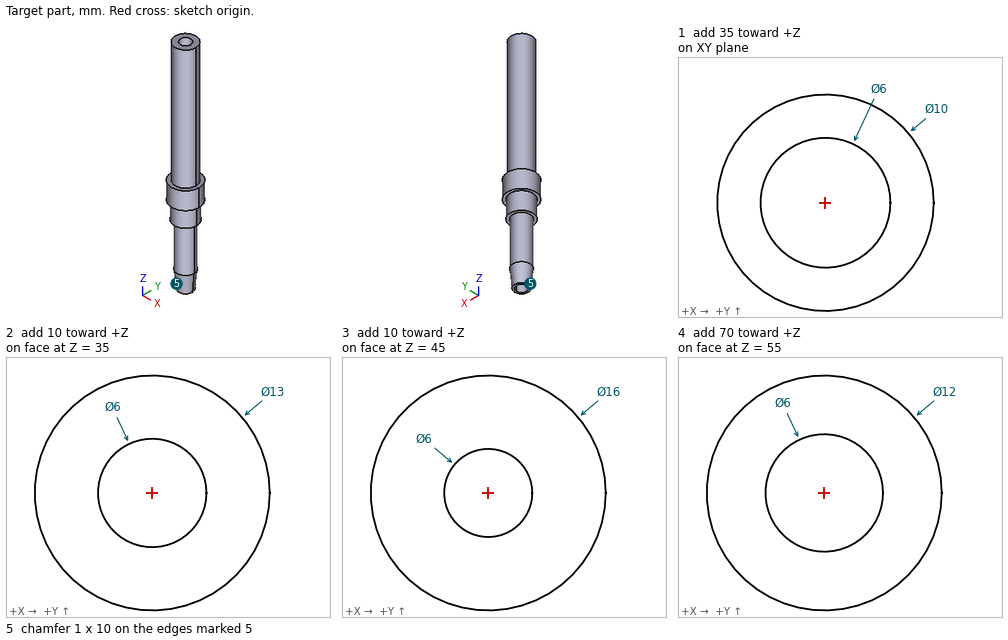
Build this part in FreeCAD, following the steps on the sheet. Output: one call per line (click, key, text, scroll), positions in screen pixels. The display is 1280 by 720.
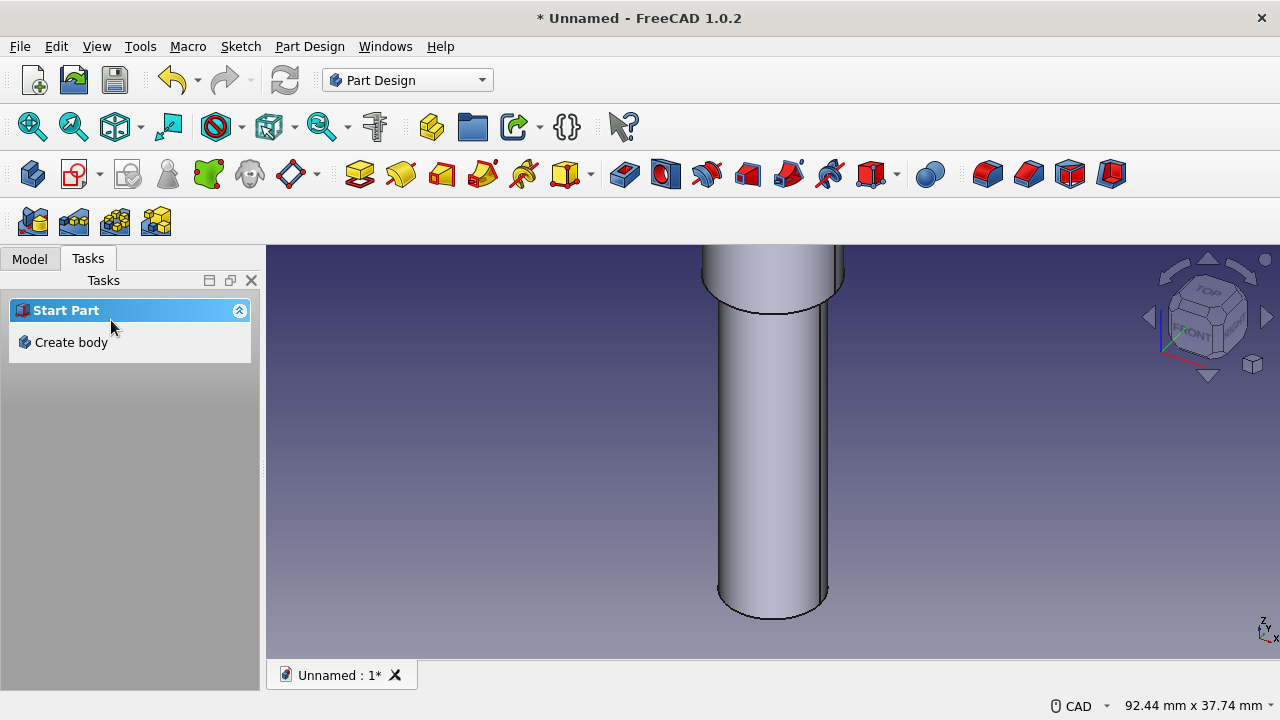
click(33, 128)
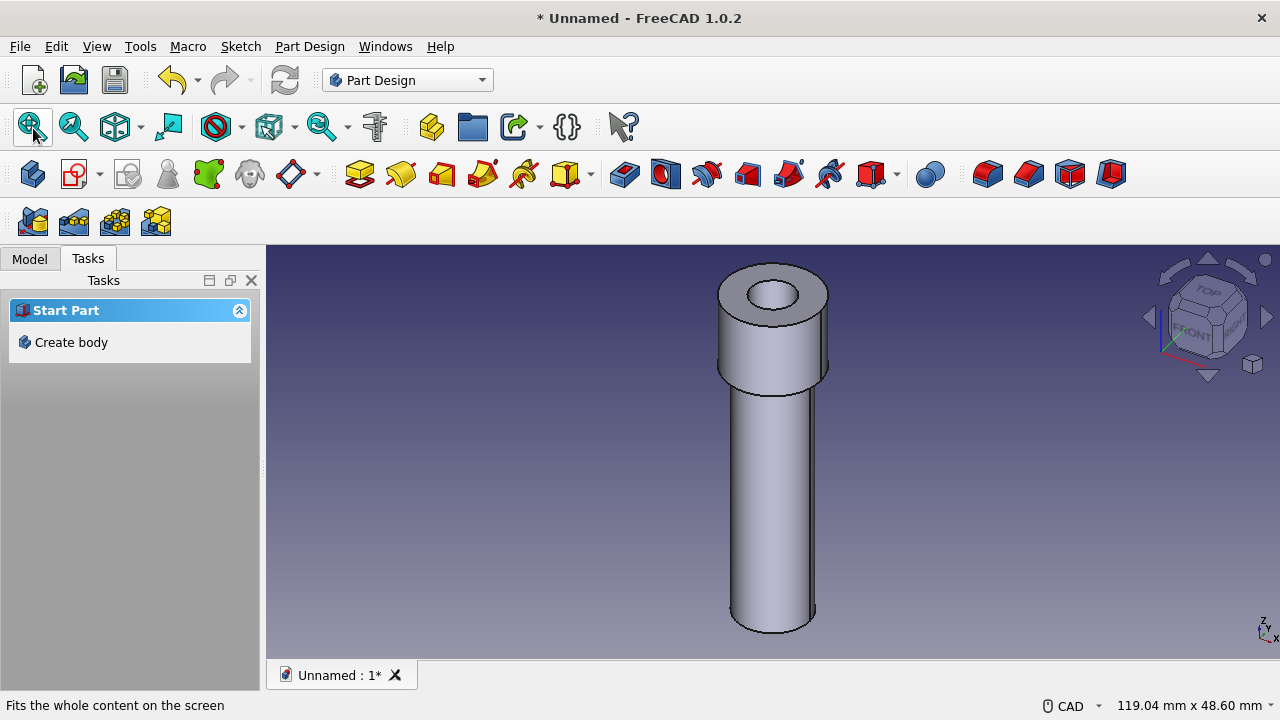
click(816, 287)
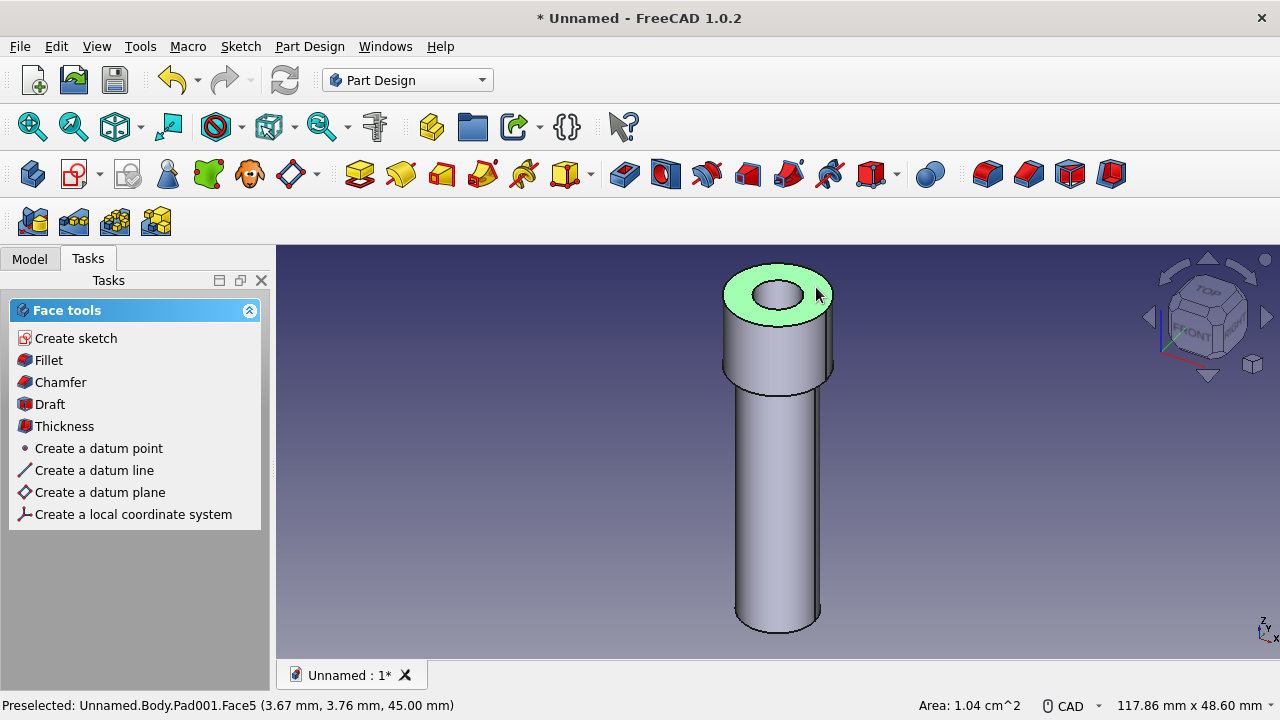
click(74, 174)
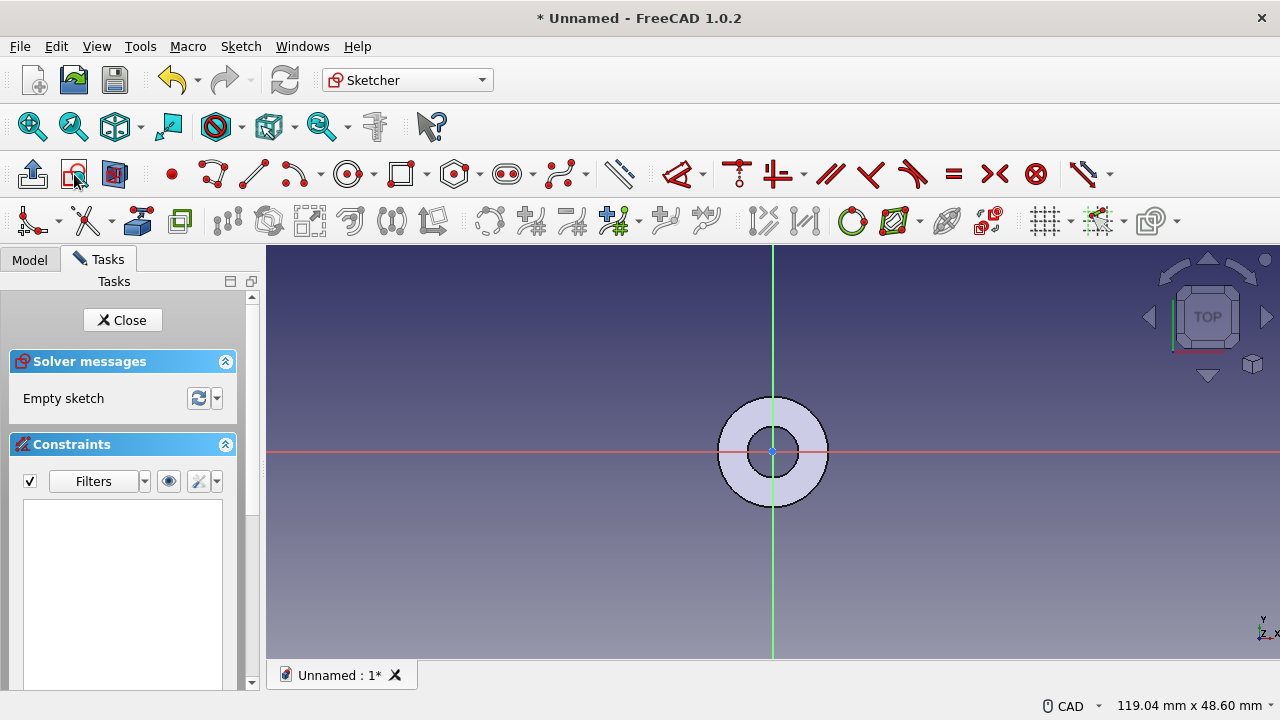
scroll(856, 452, up, 3)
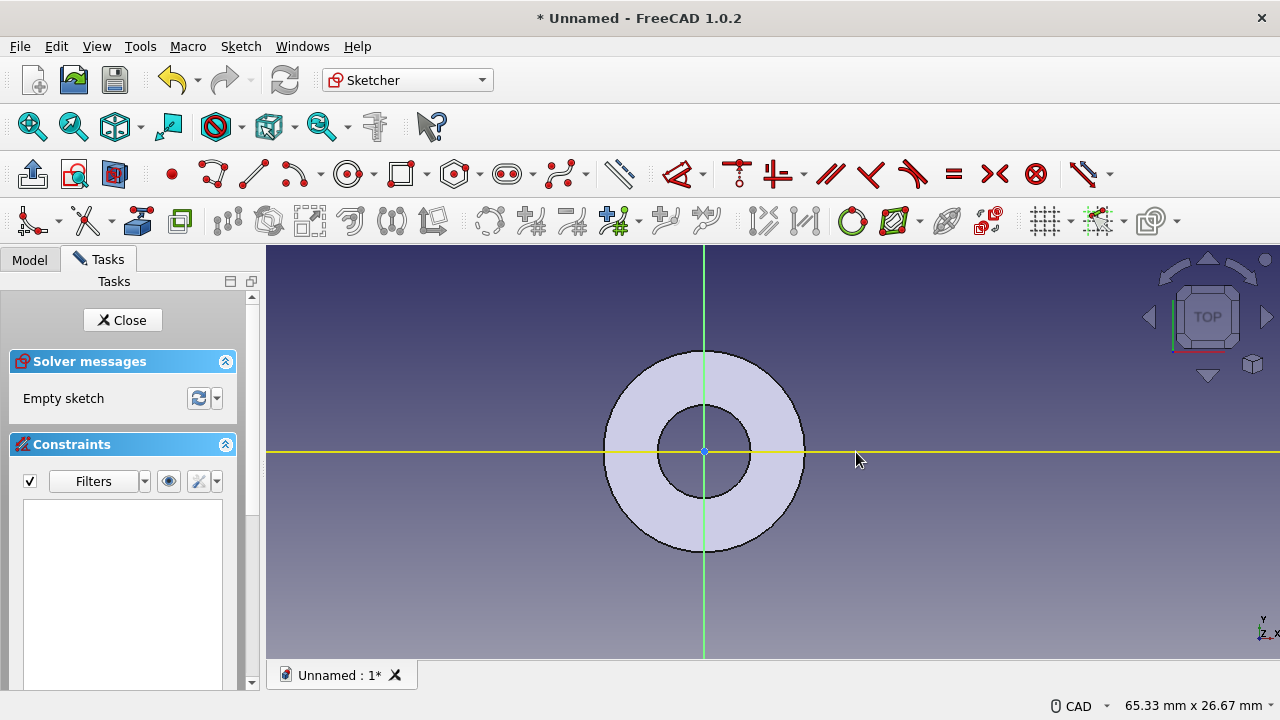
click(348, 174)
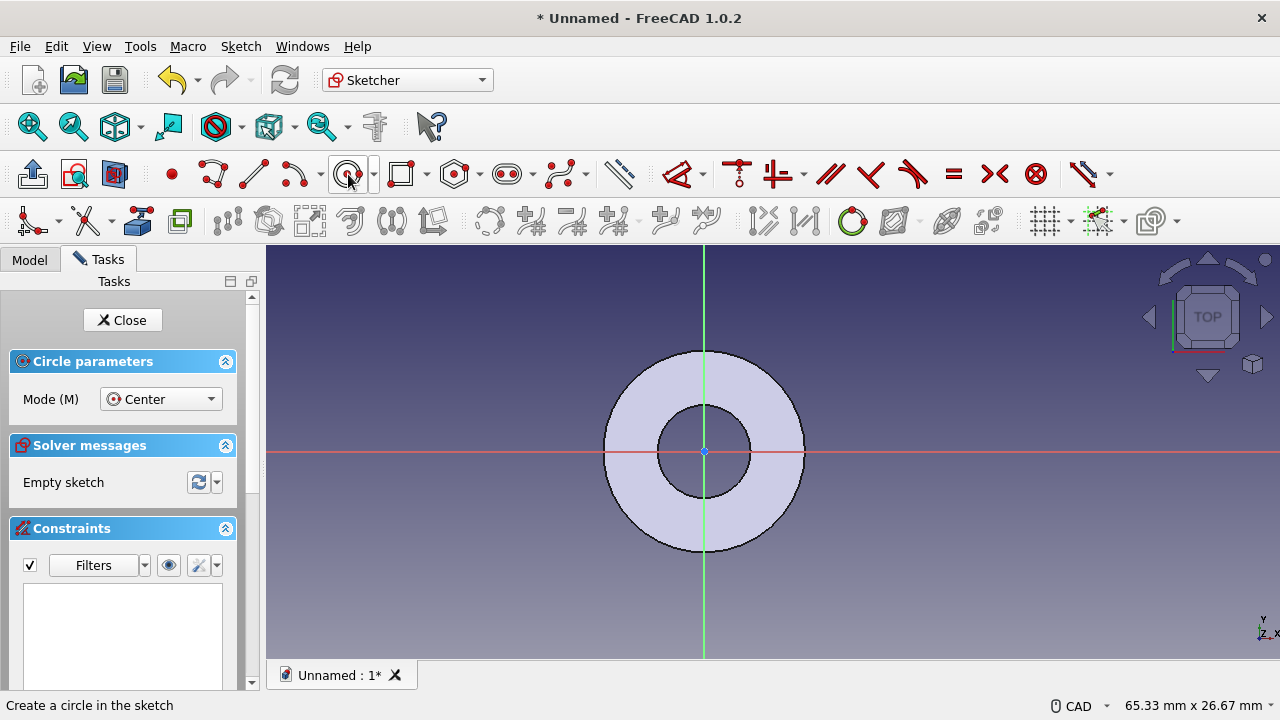
click(704, 452)
click(792, 364)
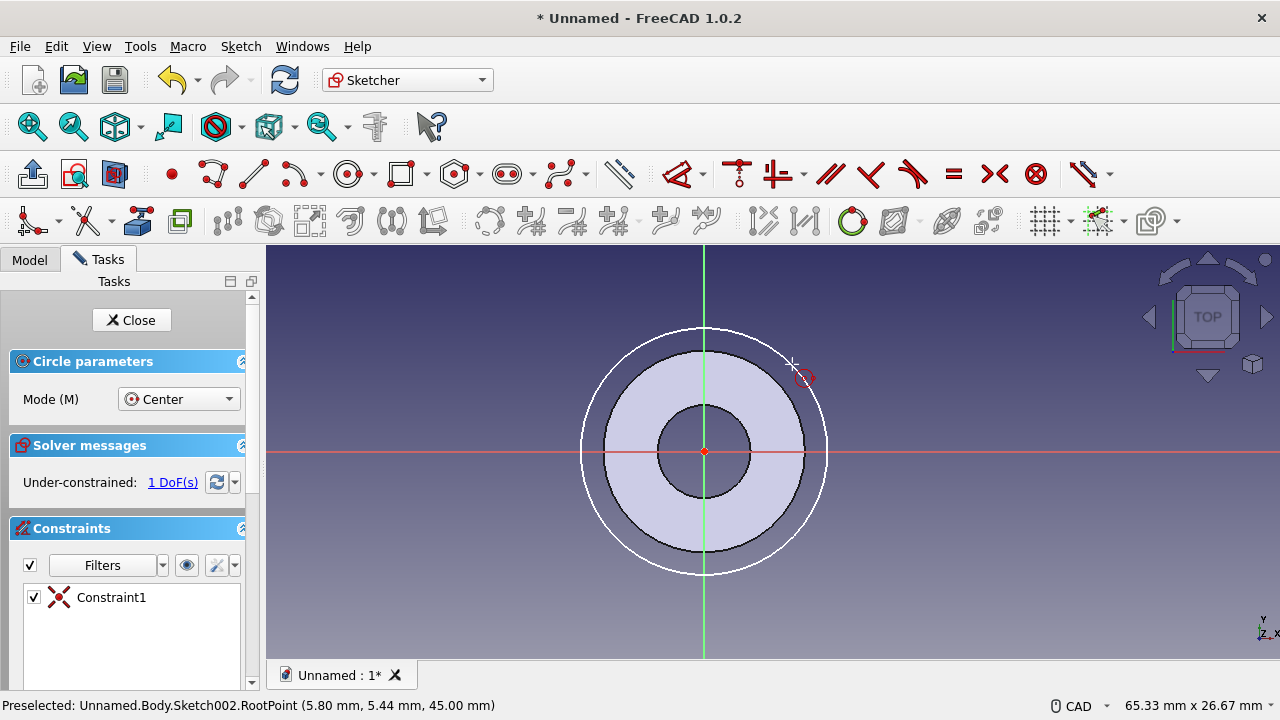
click(704, 452)
click(737, 419)
key(Escape)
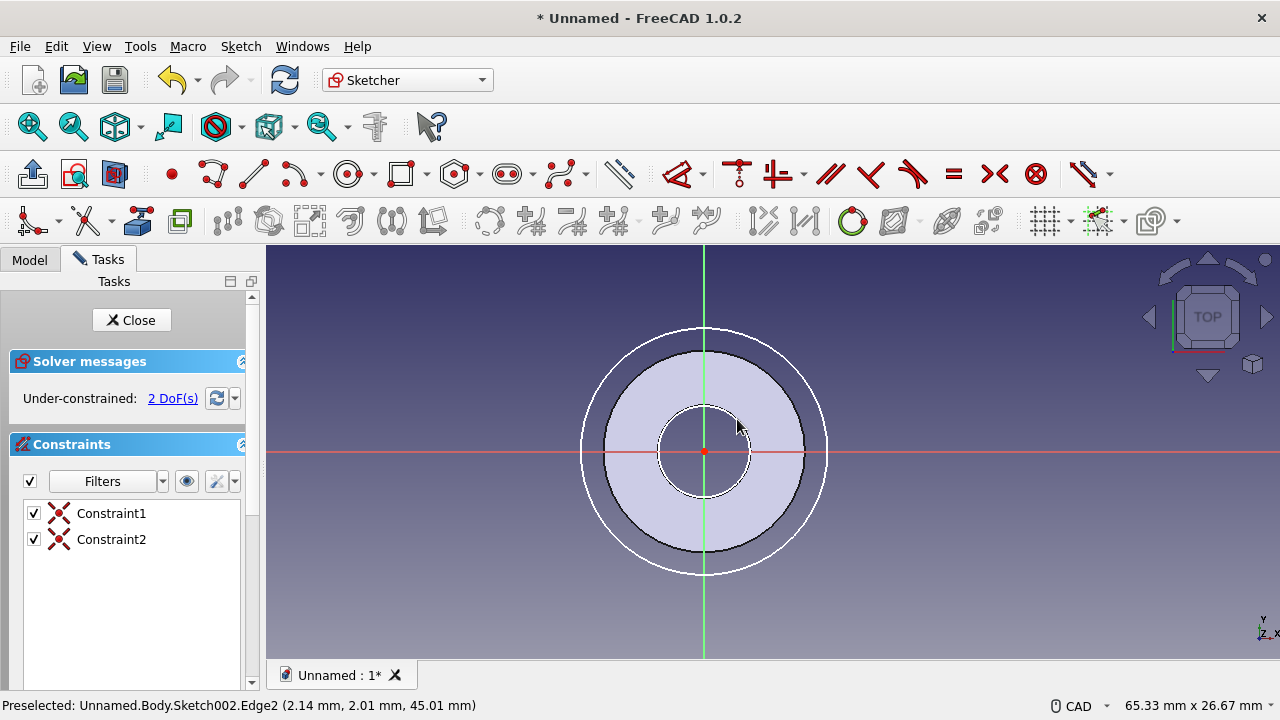
click(676, 174)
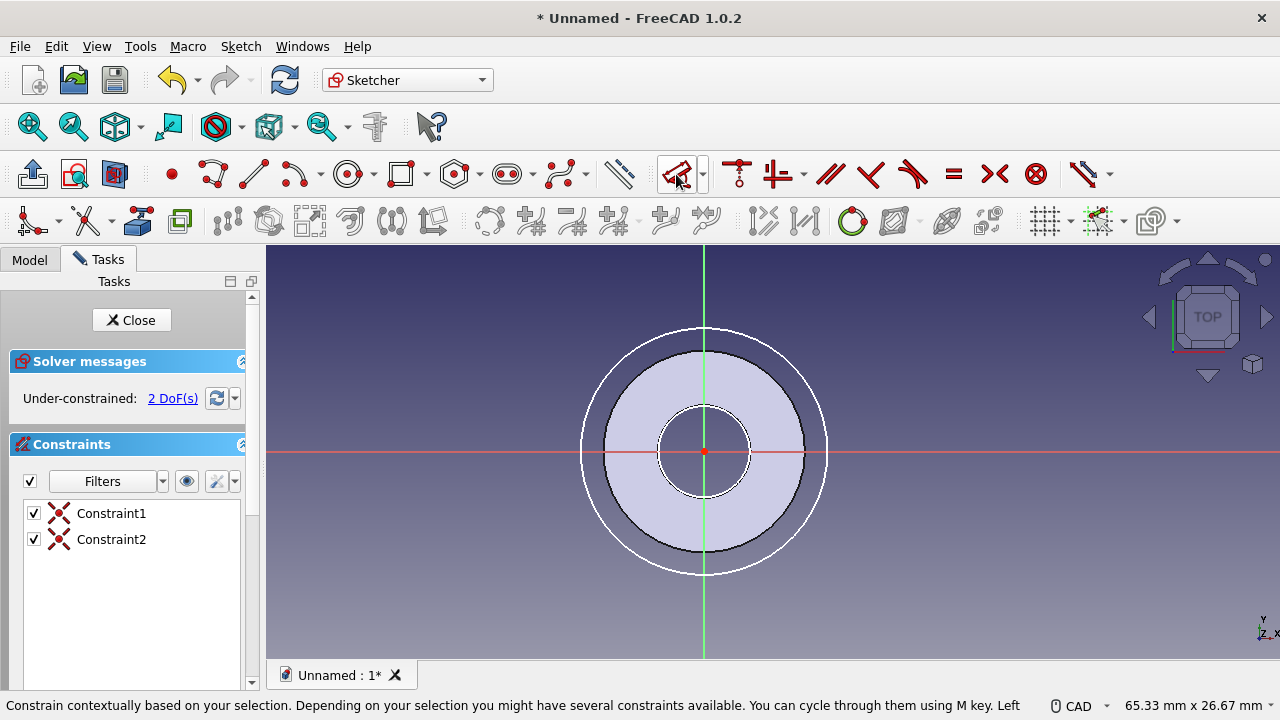
click(791, 364)
click(814, 341)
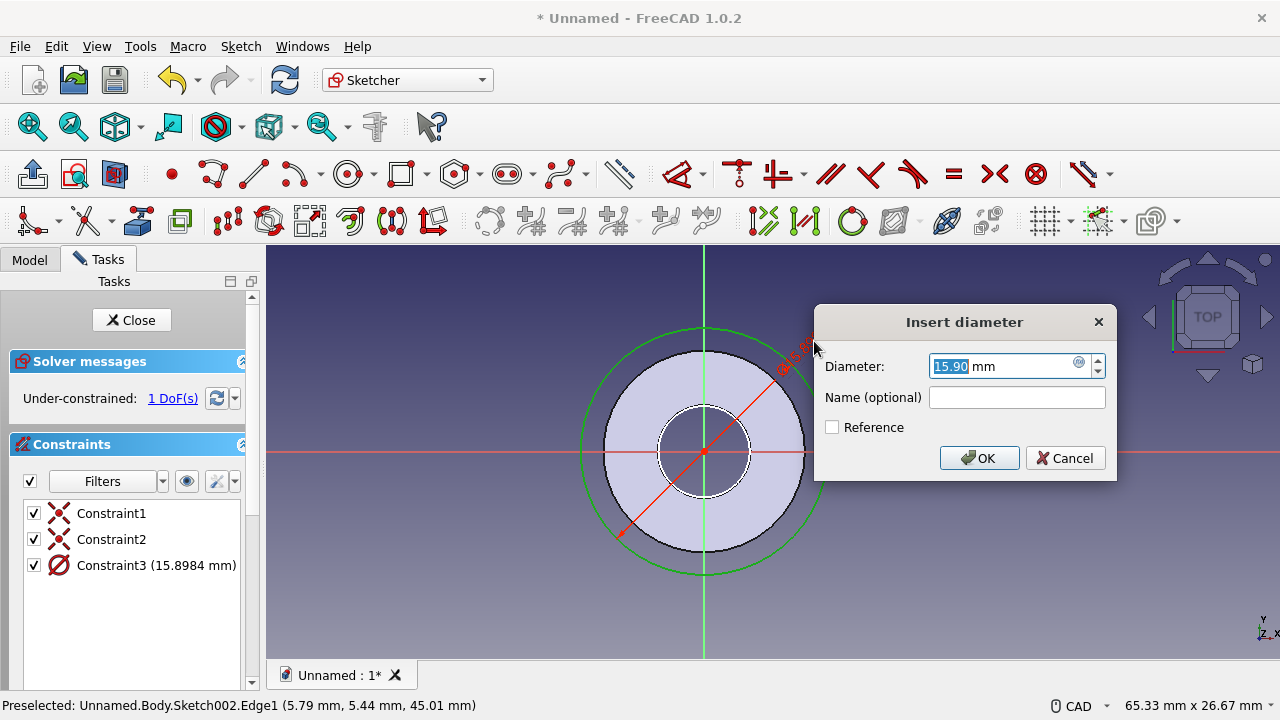
text(16)
key(Return)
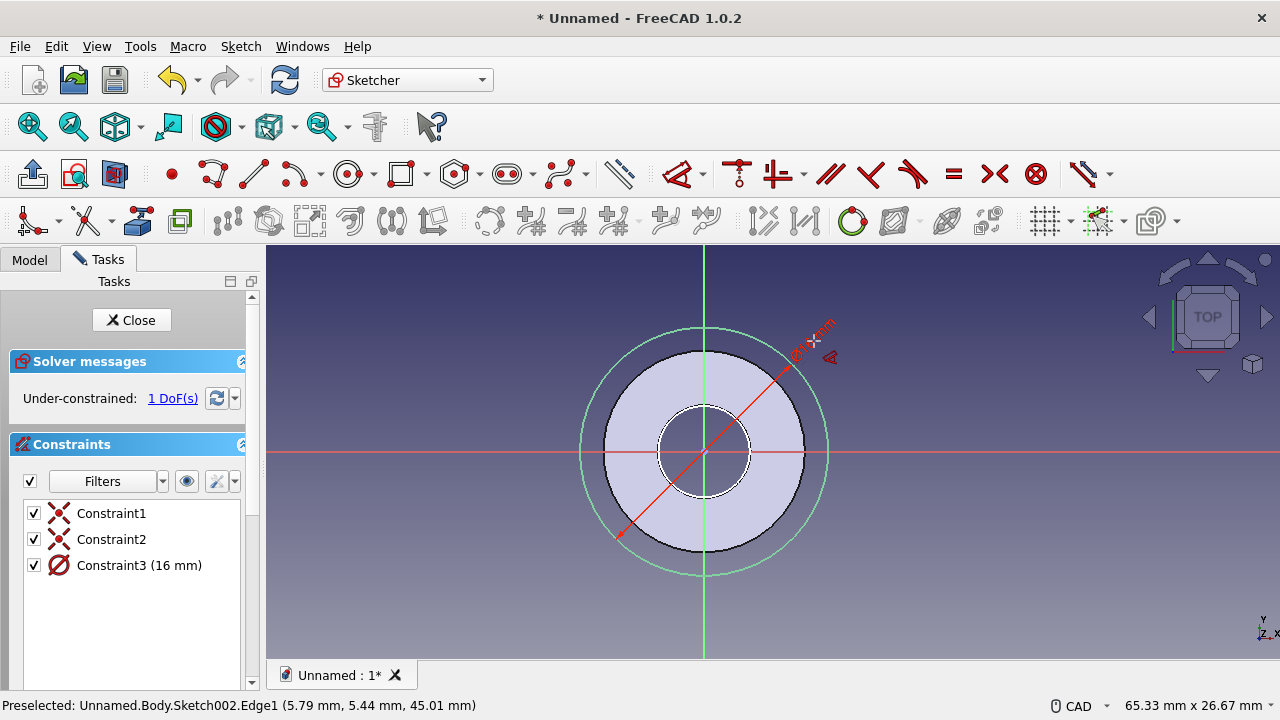
click(736, 419)
click(758, 396)